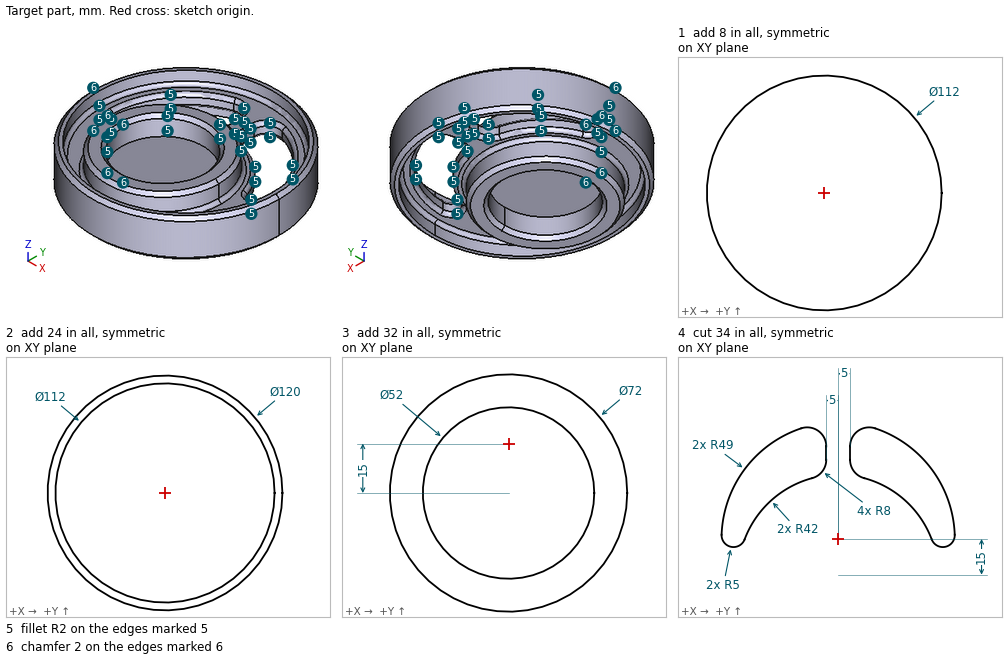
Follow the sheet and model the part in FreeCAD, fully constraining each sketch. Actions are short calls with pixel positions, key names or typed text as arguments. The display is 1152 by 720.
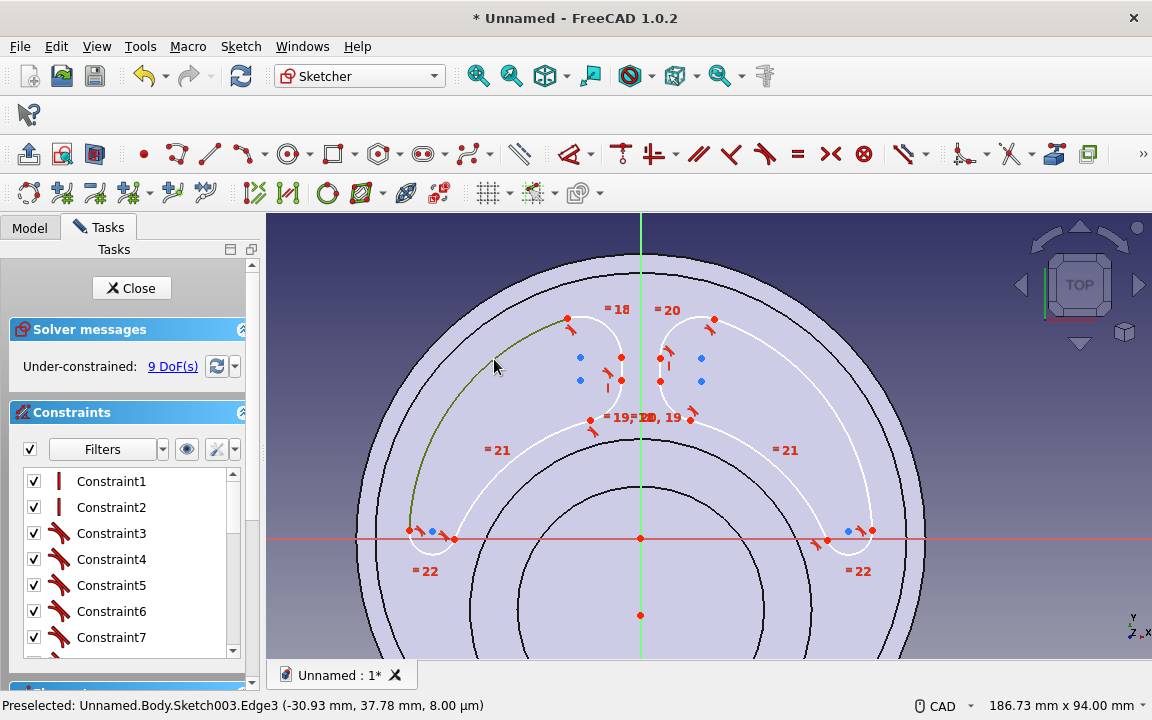
click(854, 449)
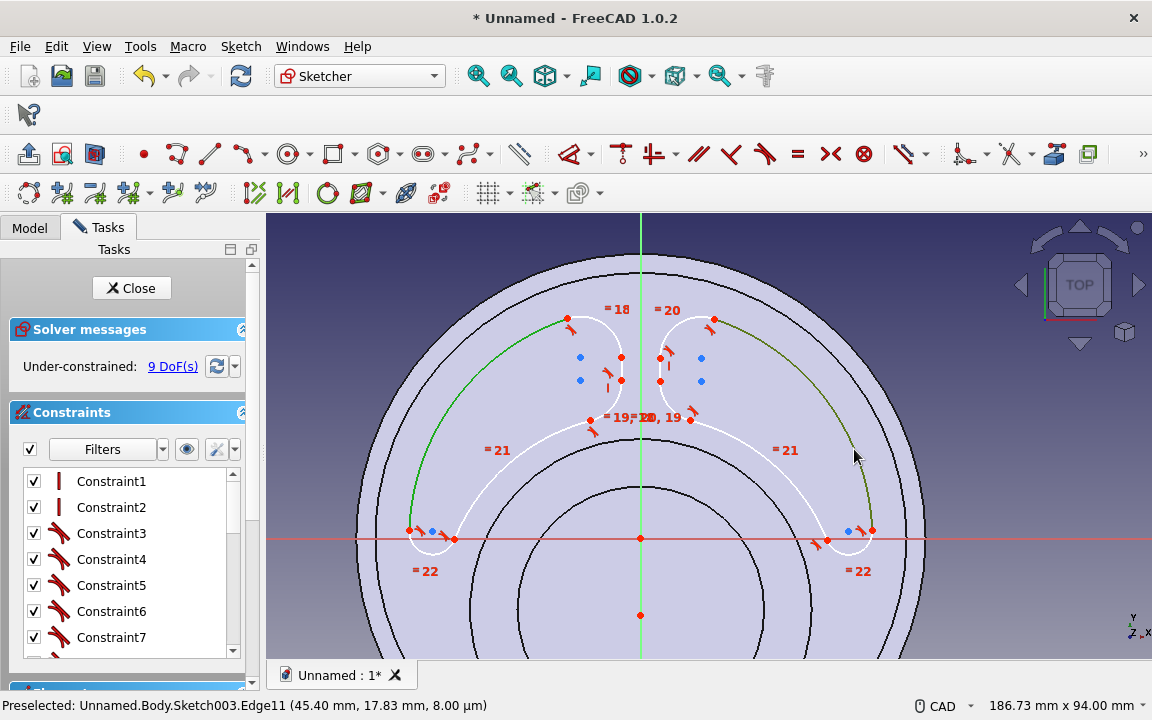
key(e)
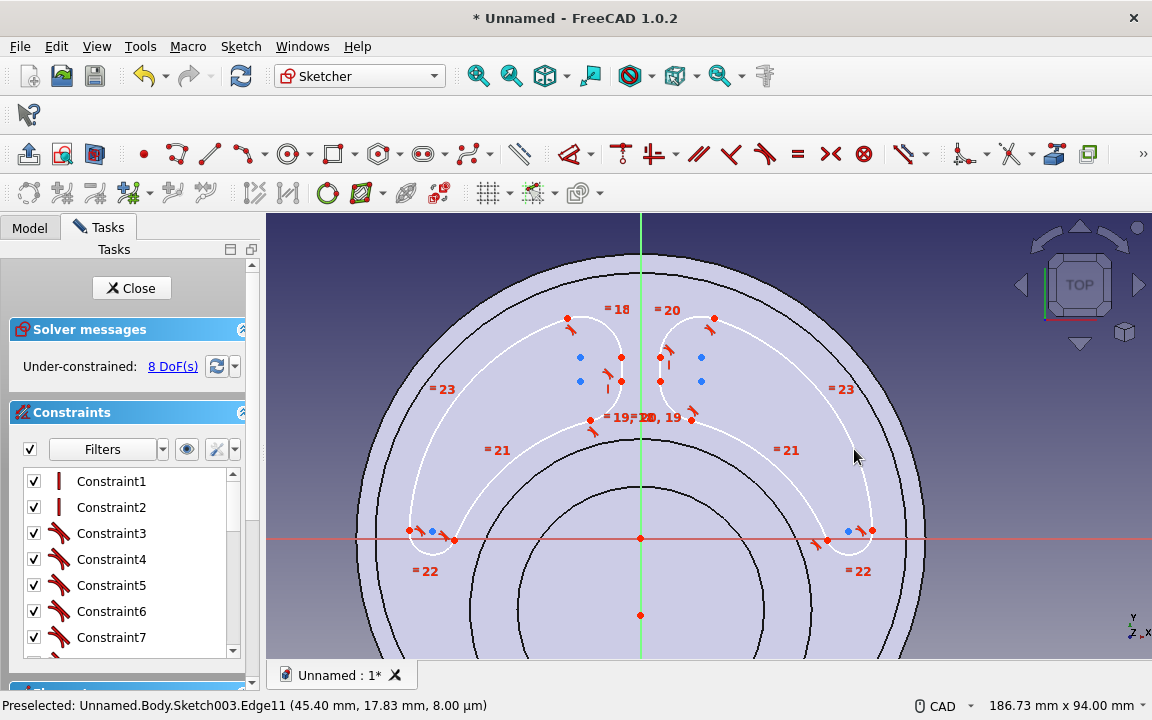
click(641, 616)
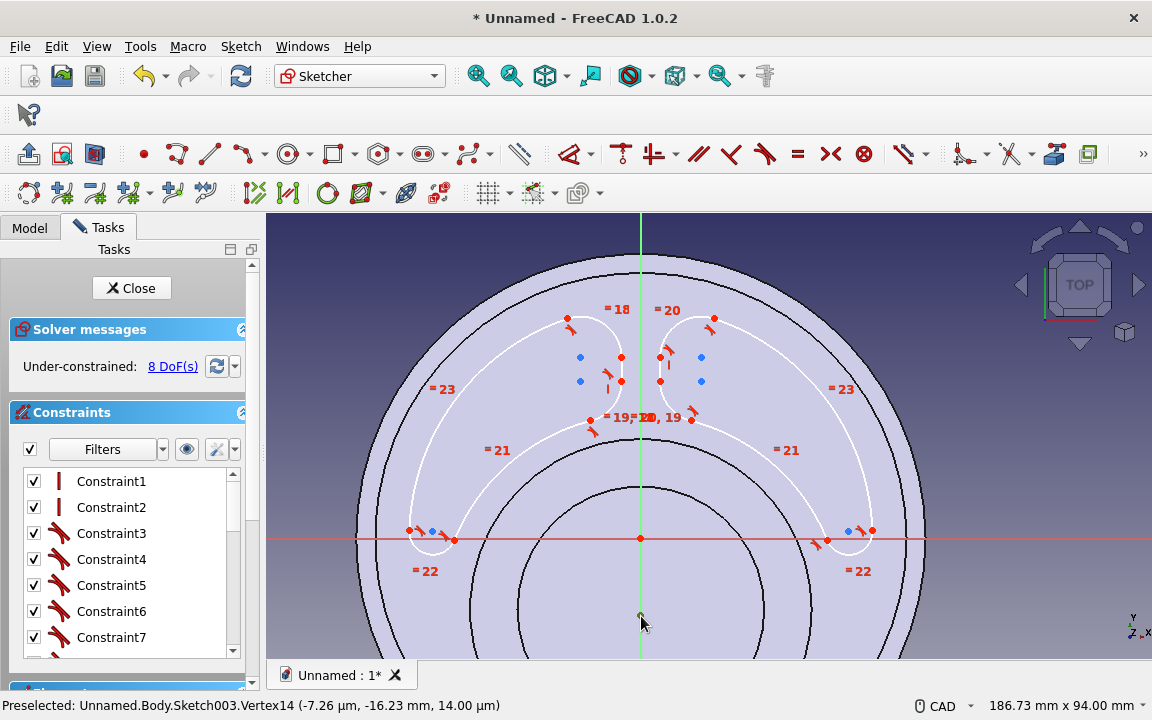
click(641, 603)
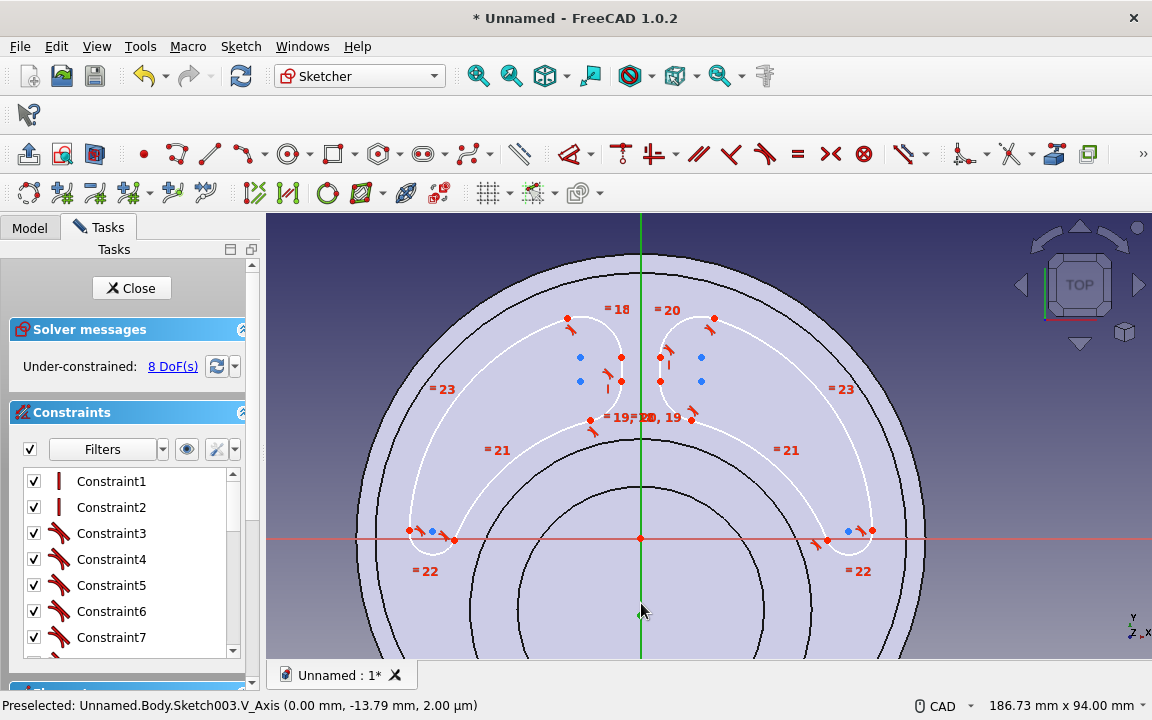
key(c)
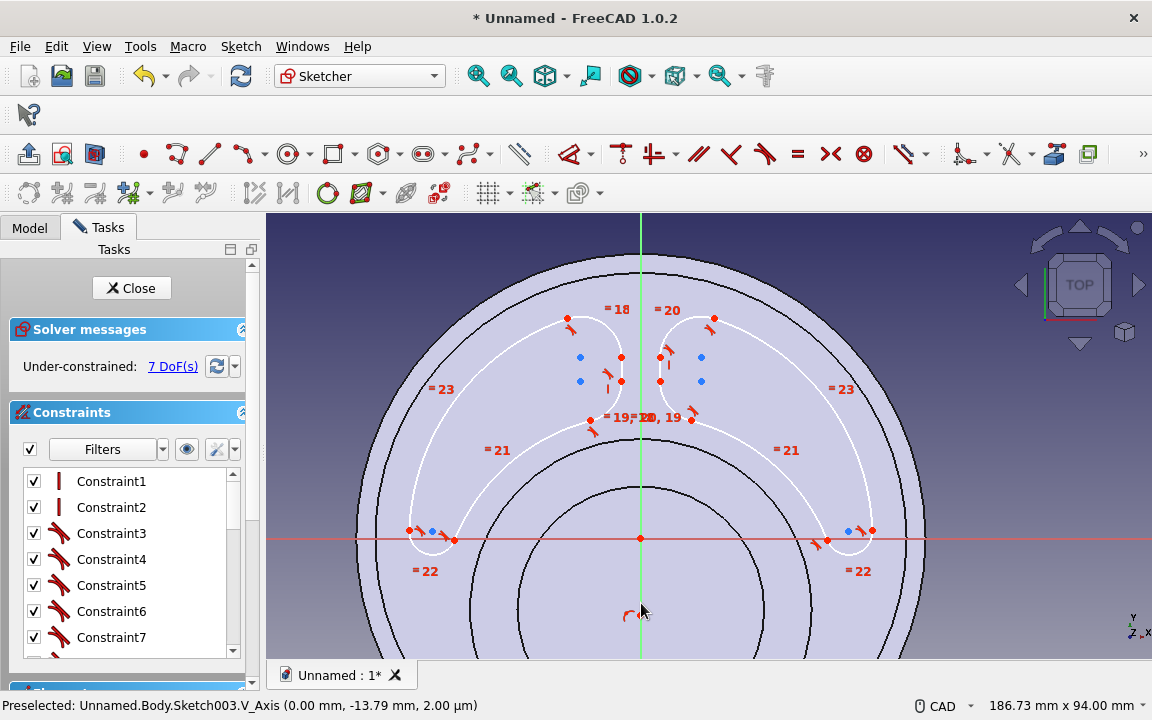
click(568, 154)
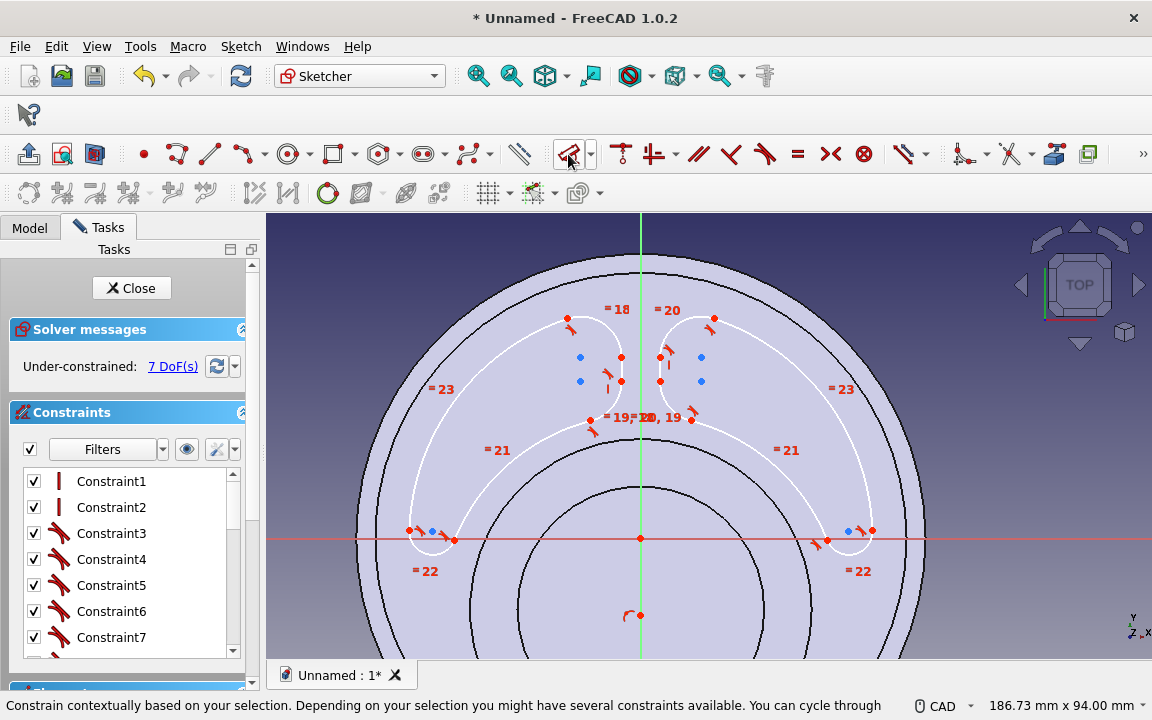
click(615, 336)
click(616, 294)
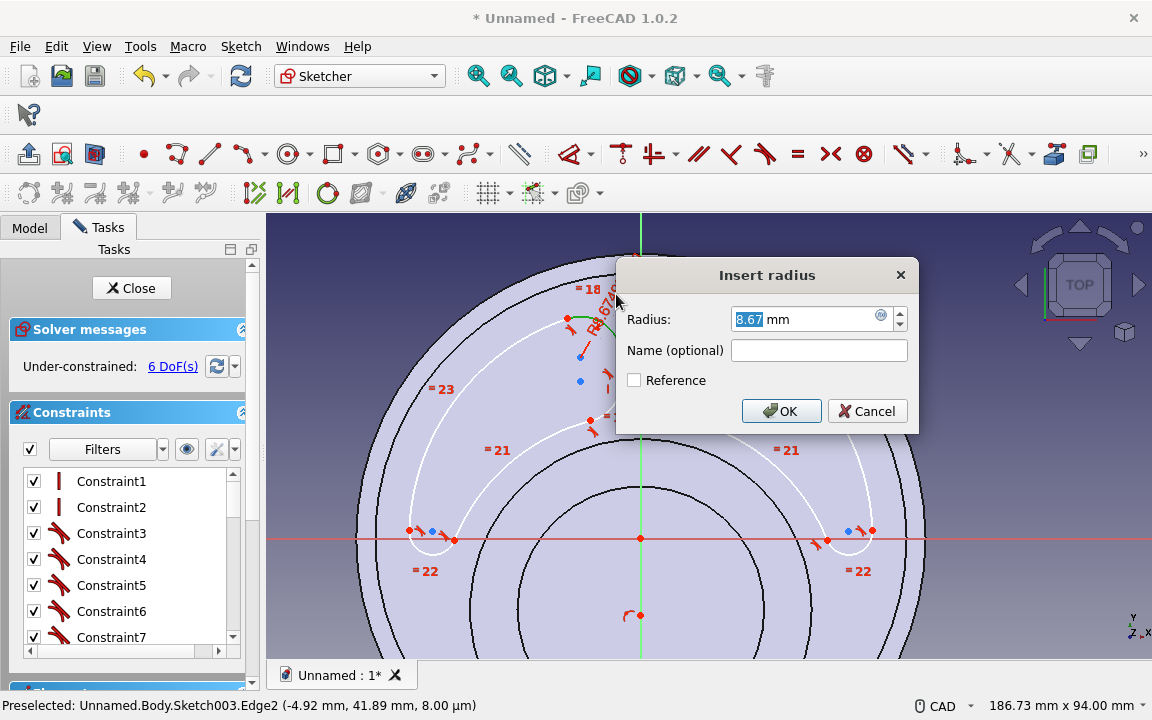
text(8)
key(Return)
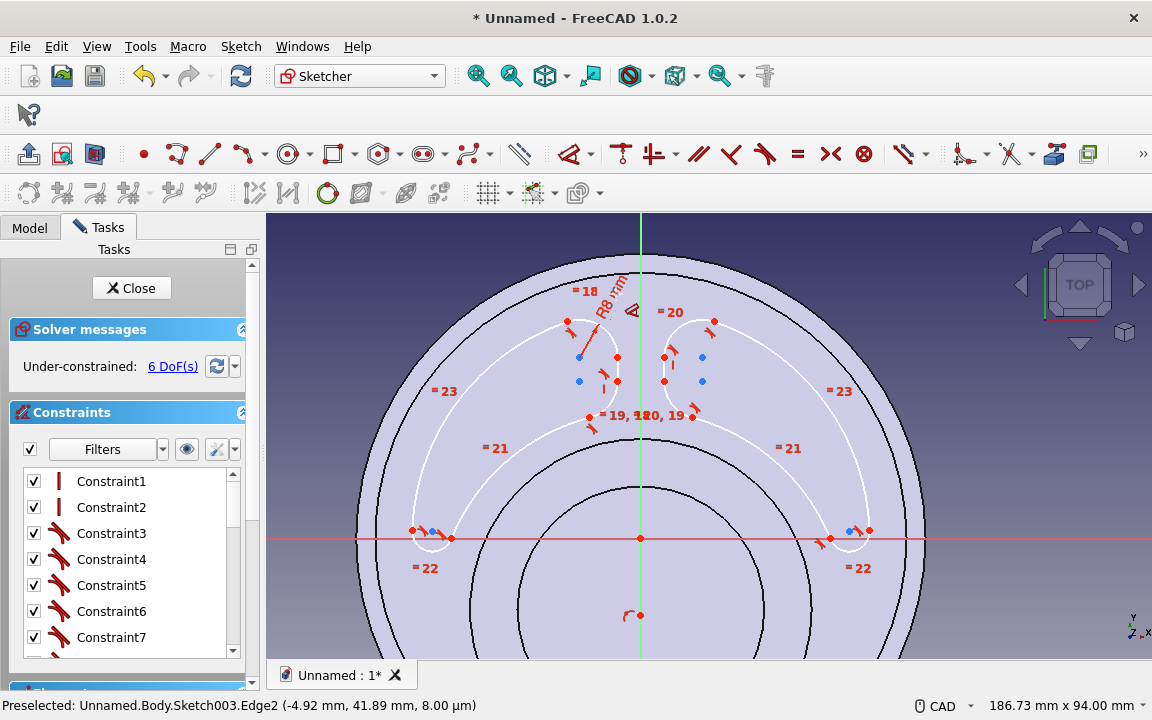
click(495, 362)
click(475, 337)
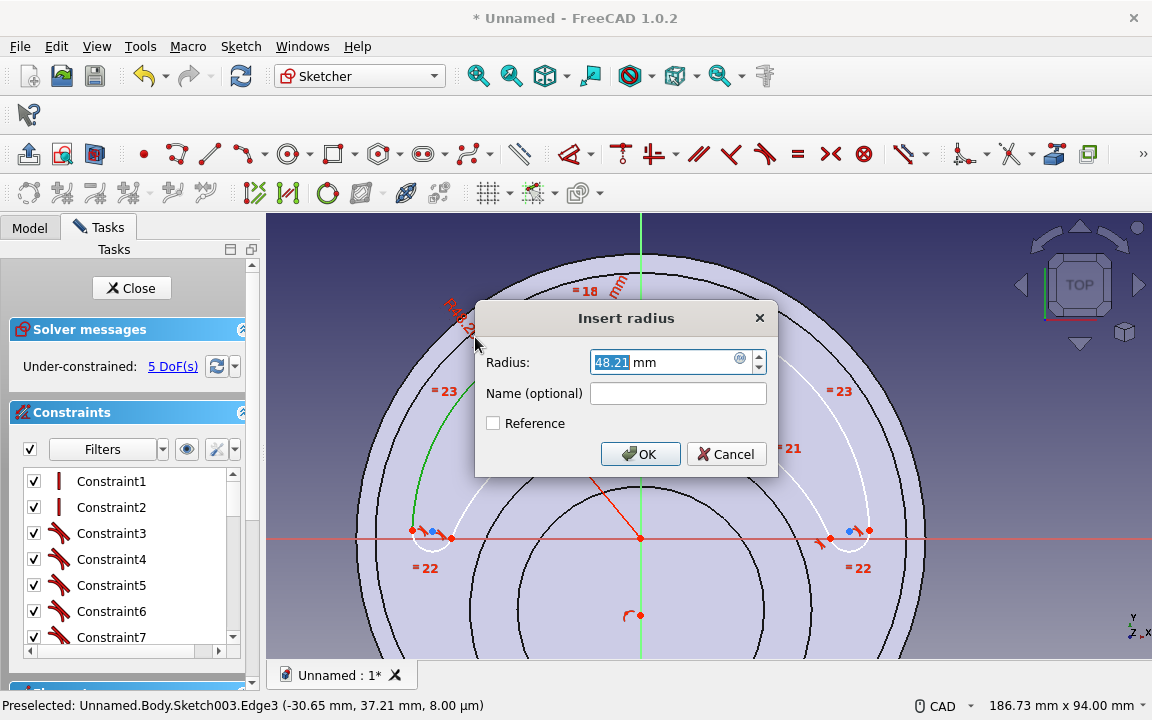
text(49)
key(Return)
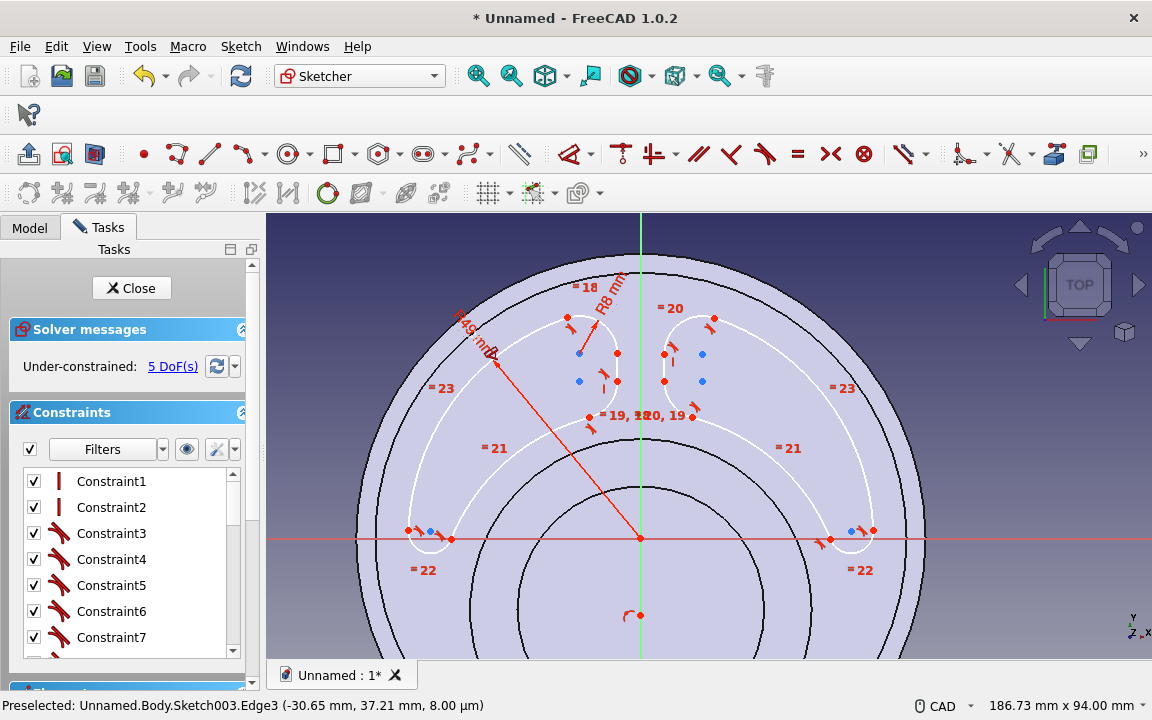
scroll(438, 552, up, 3)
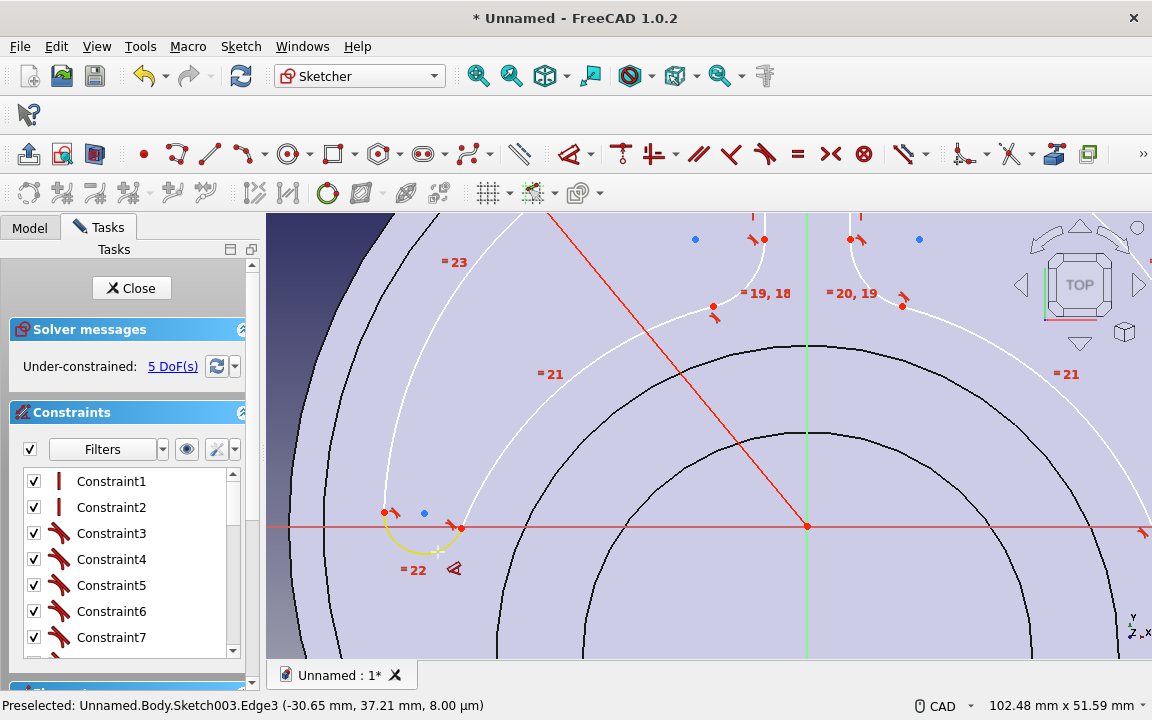
click(438, 551)
click(449, 581)